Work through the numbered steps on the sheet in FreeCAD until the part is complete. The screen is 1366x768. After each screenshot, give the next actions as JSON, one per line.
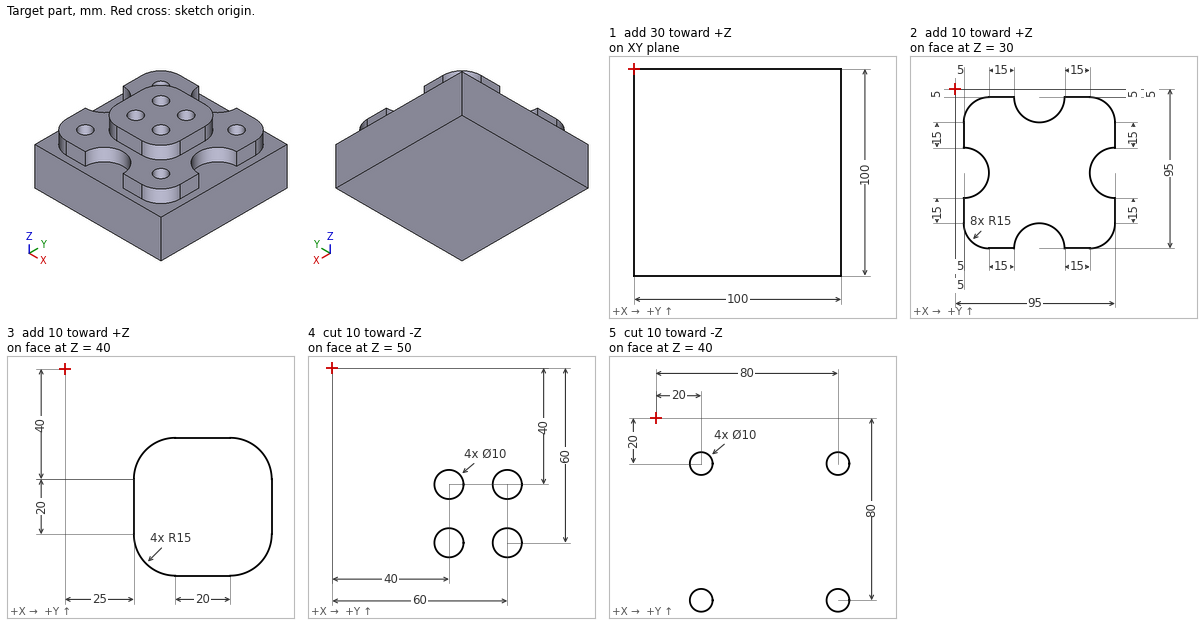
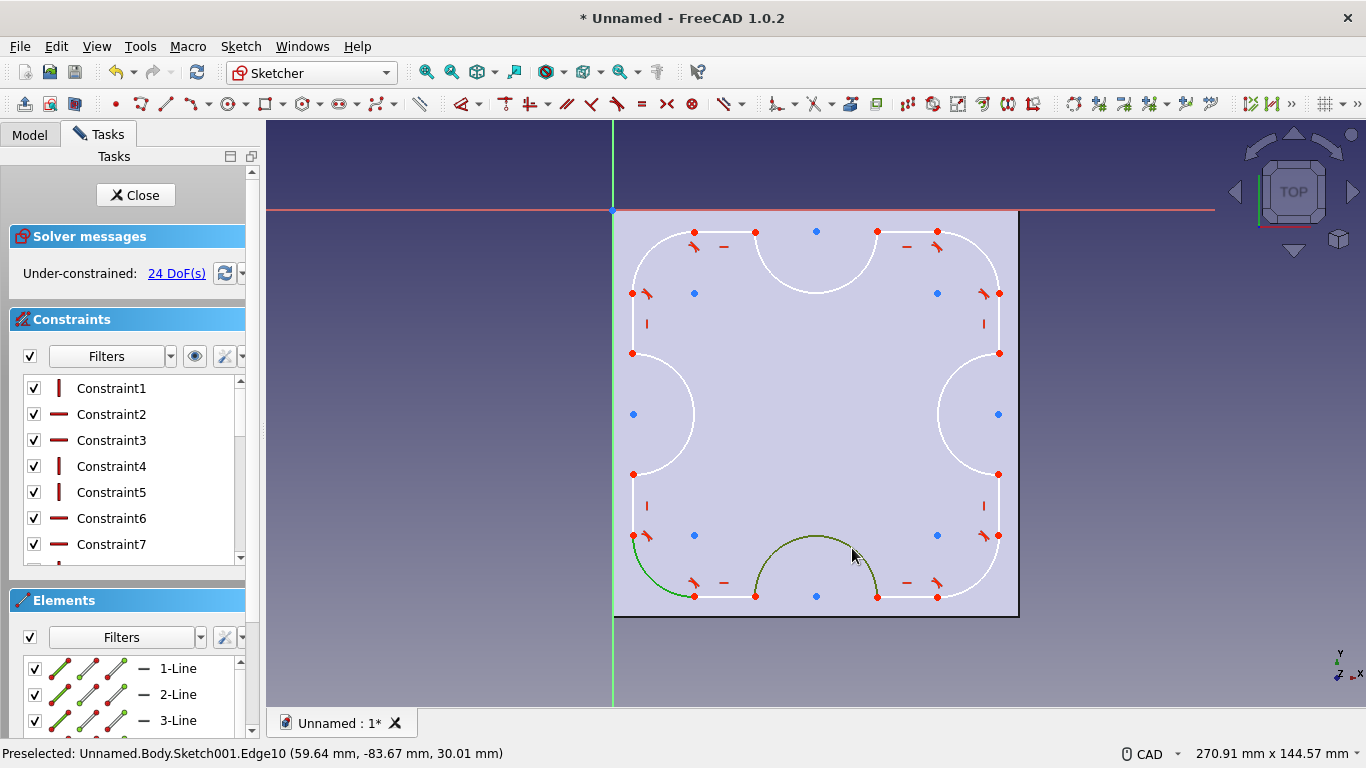
{"action": "left_click", "coordinate": [965, 591]}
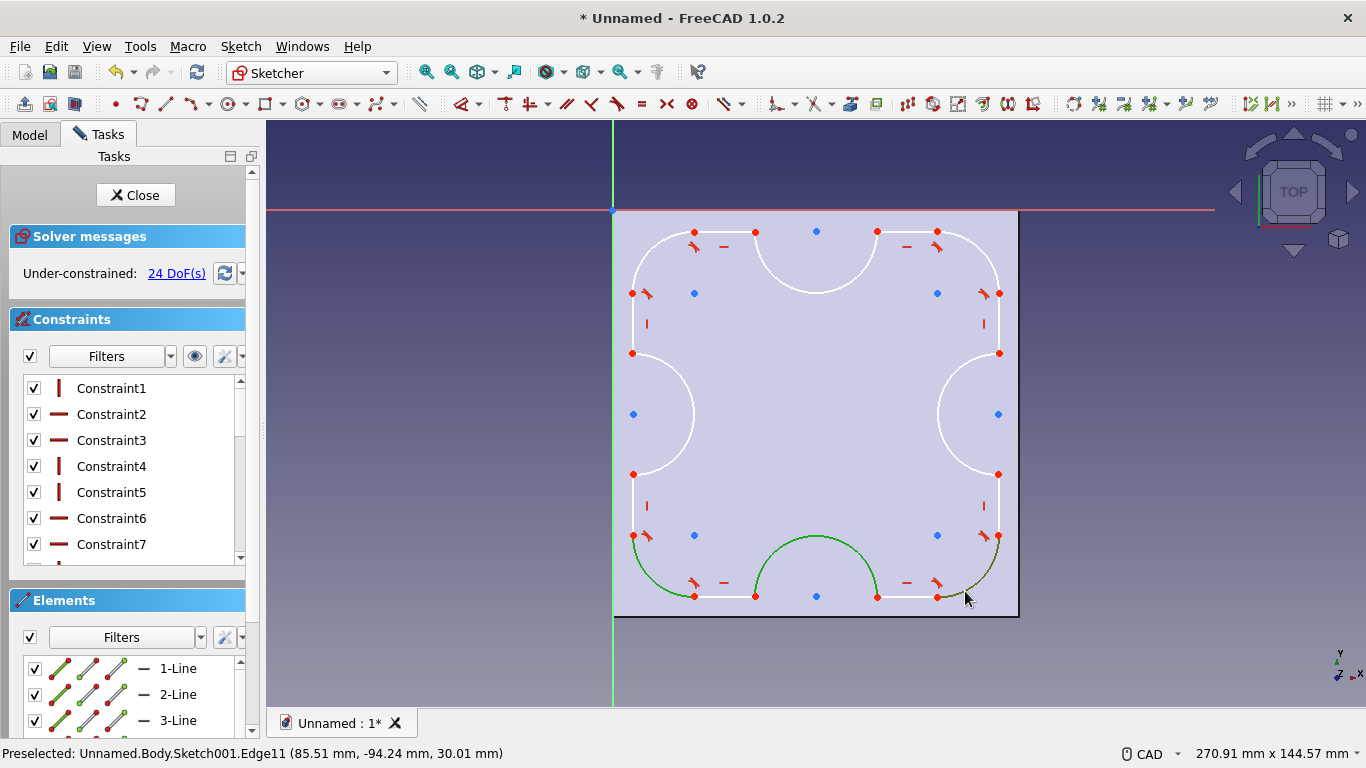
{"action": "left_click", "coordinate": [950, 379]}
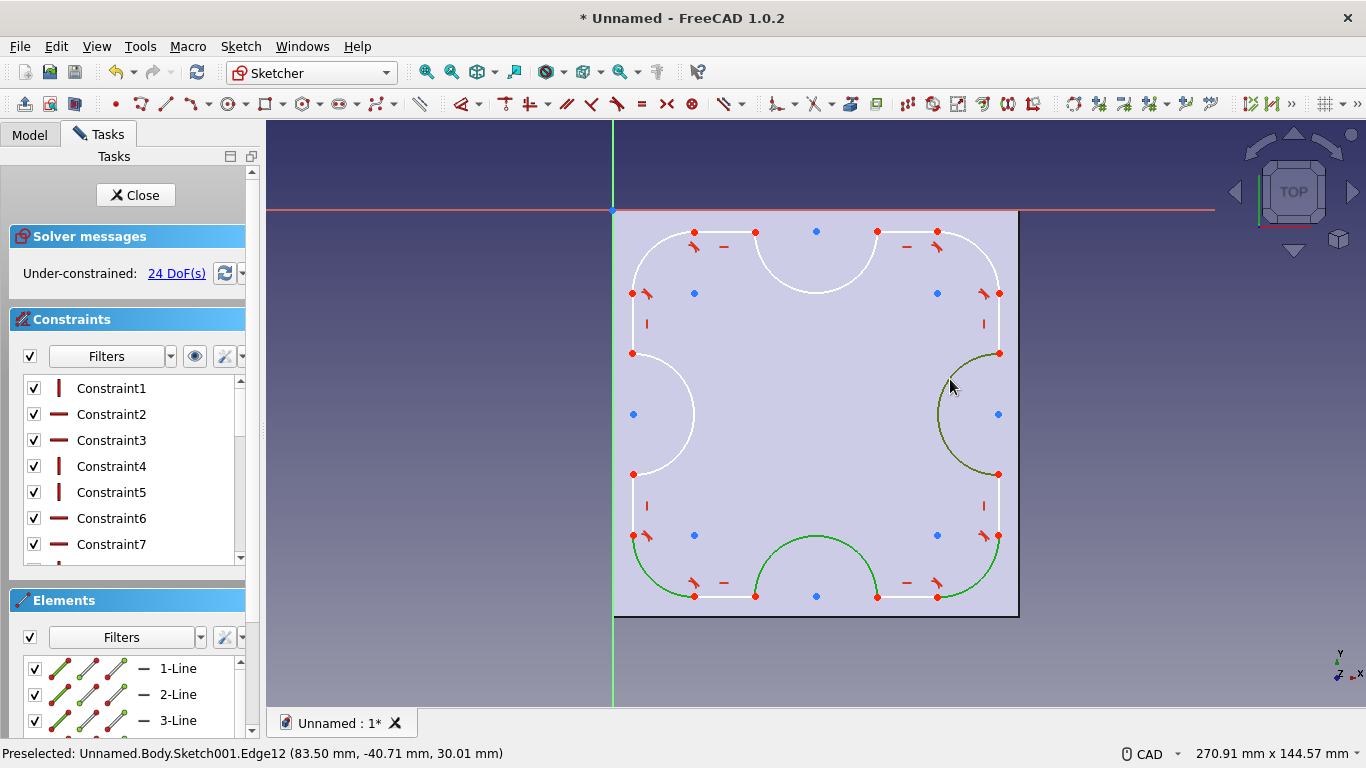
{"action": "left_click", "coordinate": [992, 266]}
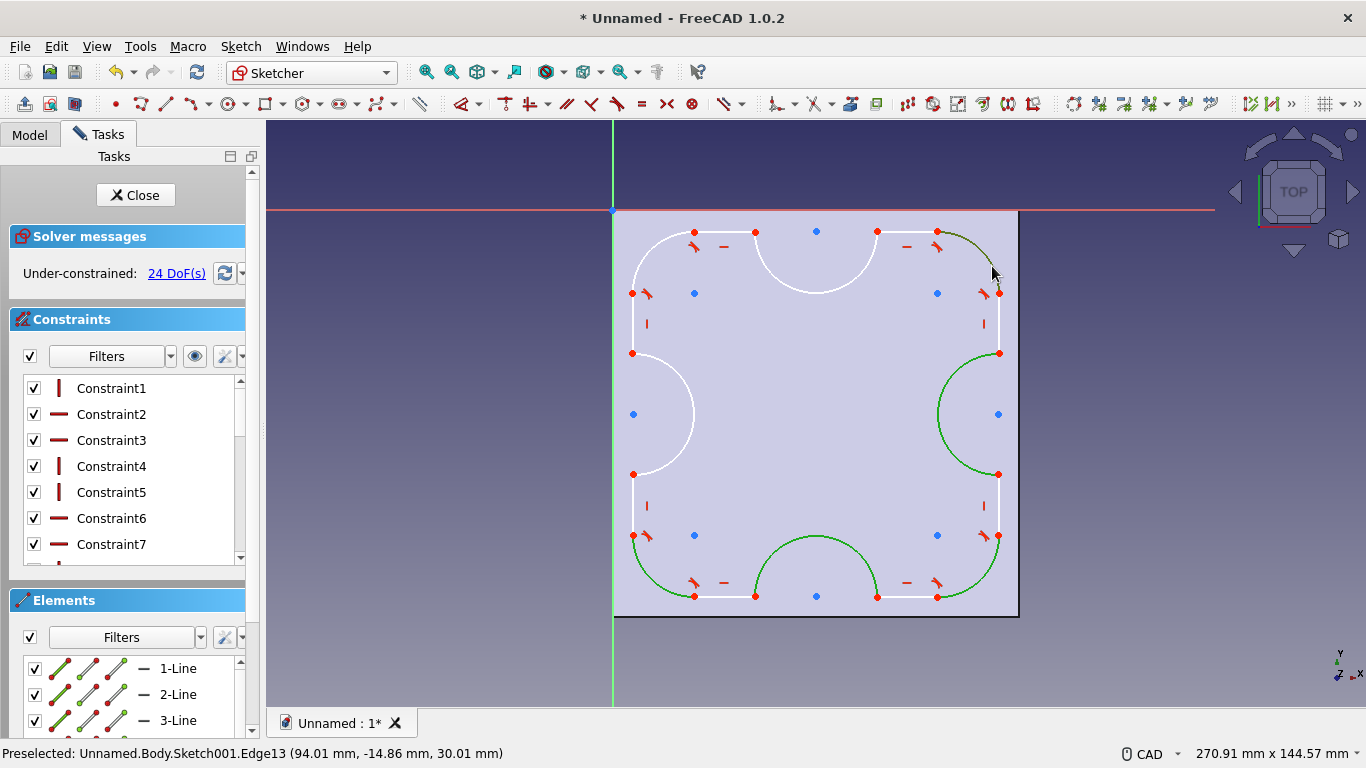
{"action": "left_click", "coordinate": [780, 281]}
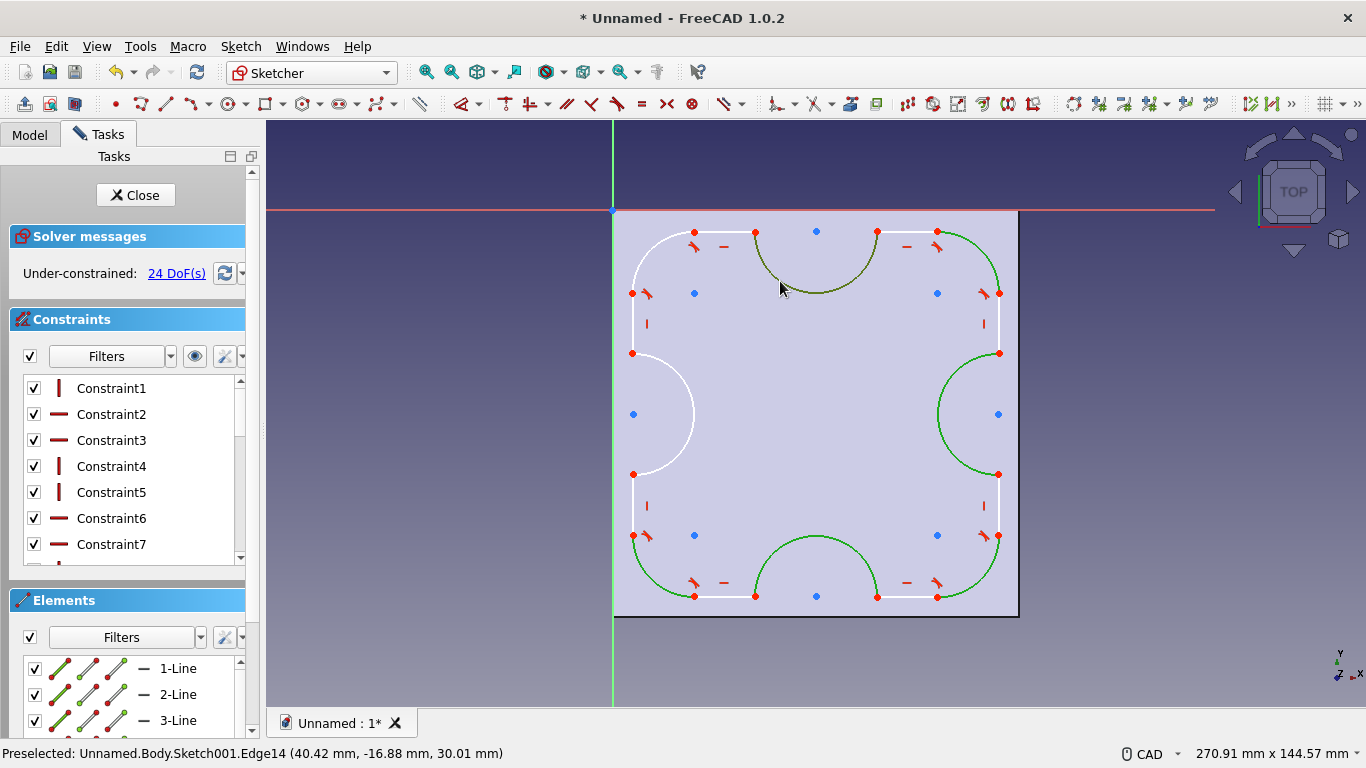
{"action": "left_click", "coordinate": [666, 239]}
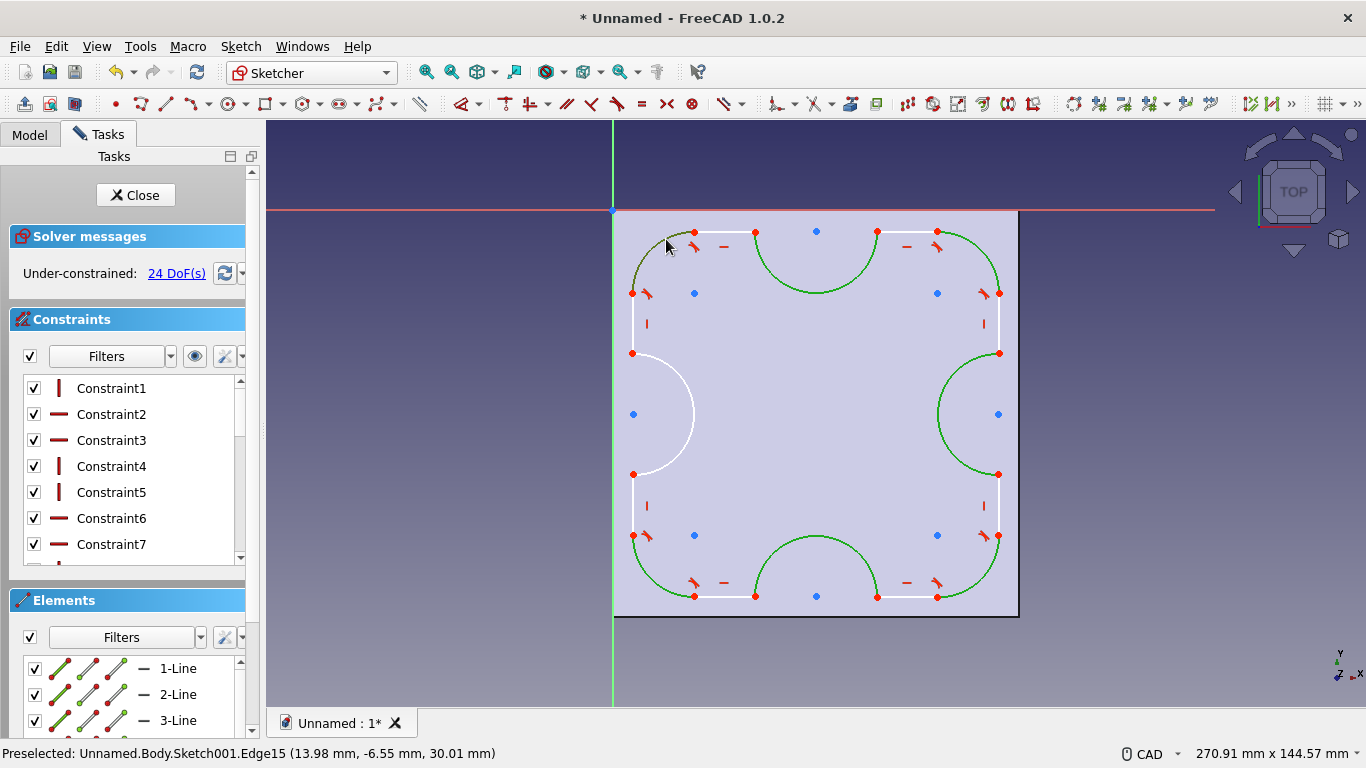
{"action": "left_click", "coordinate": [682, 450]}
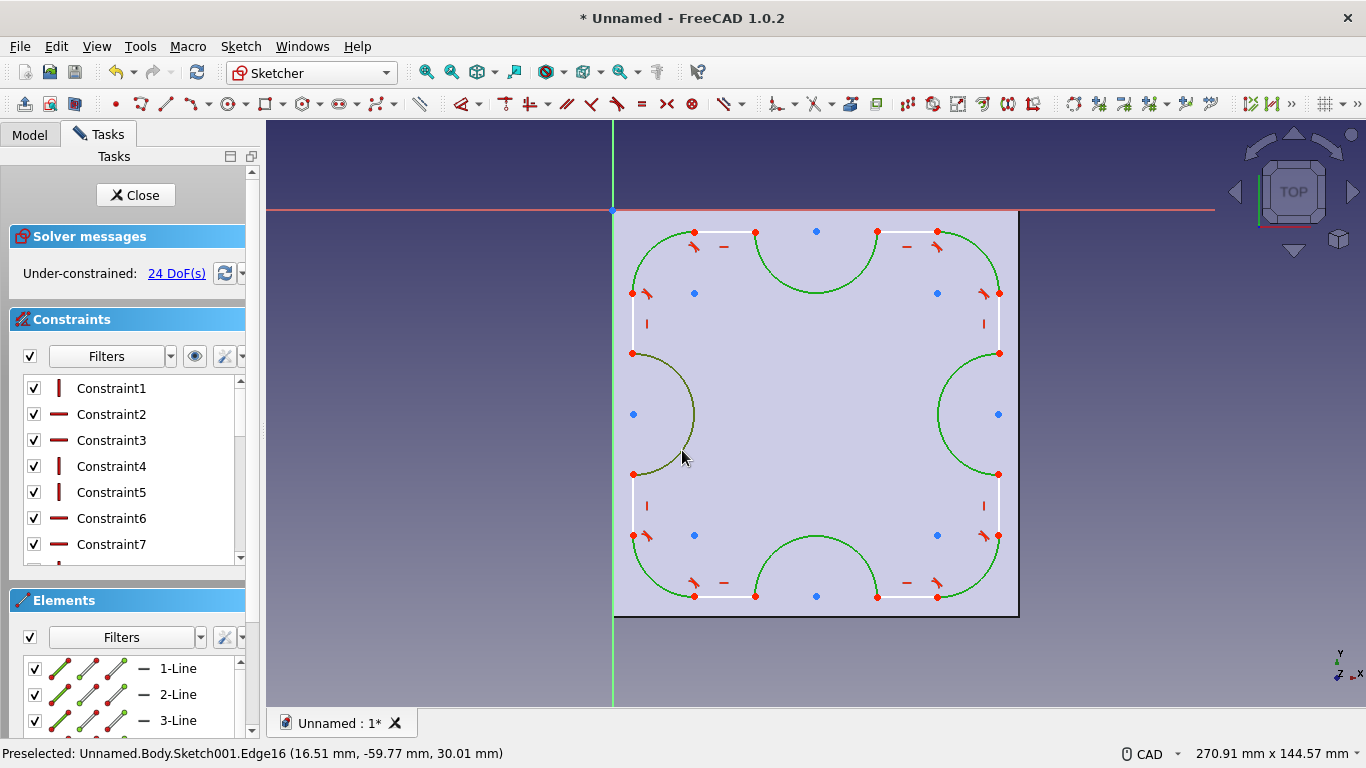
{"action": "left_click", "coordinate": [642, 104]}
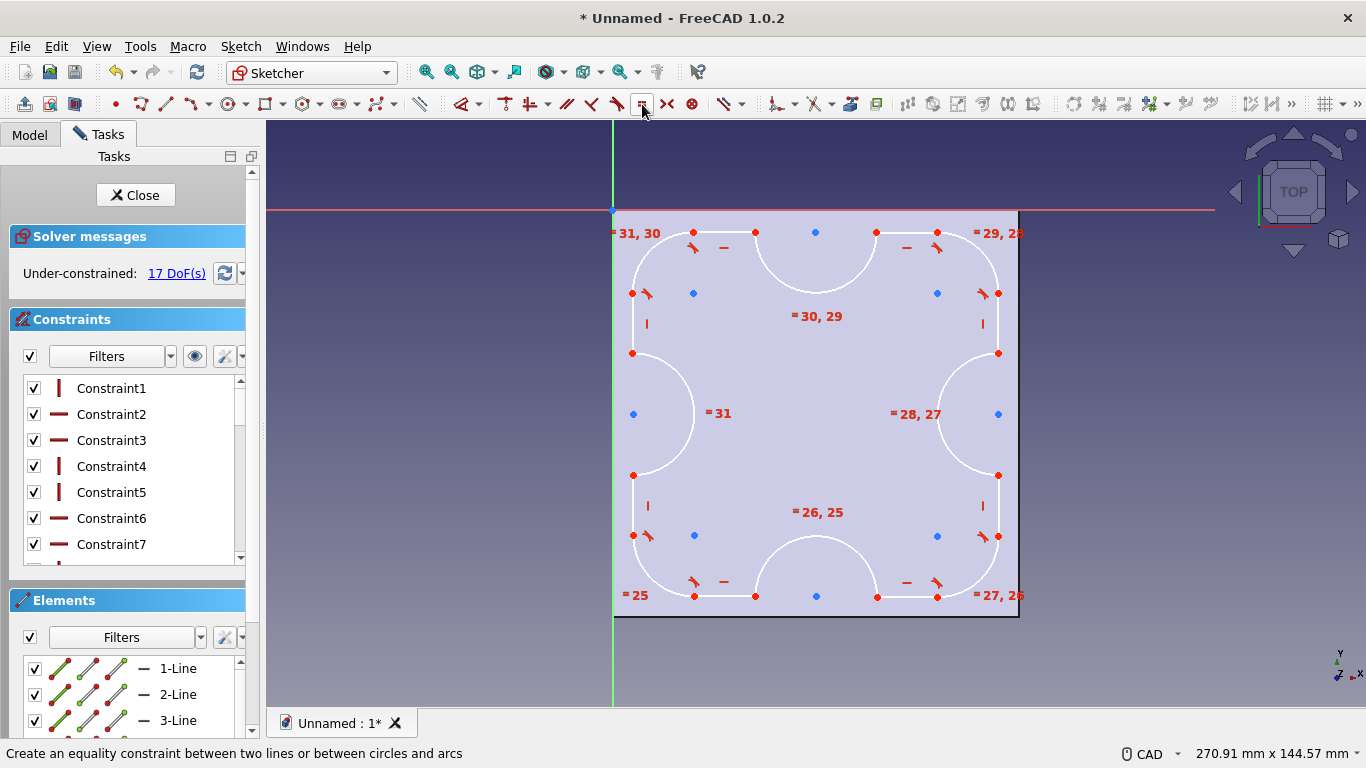
{"action": "left_click", "coordinate": [460, 104]}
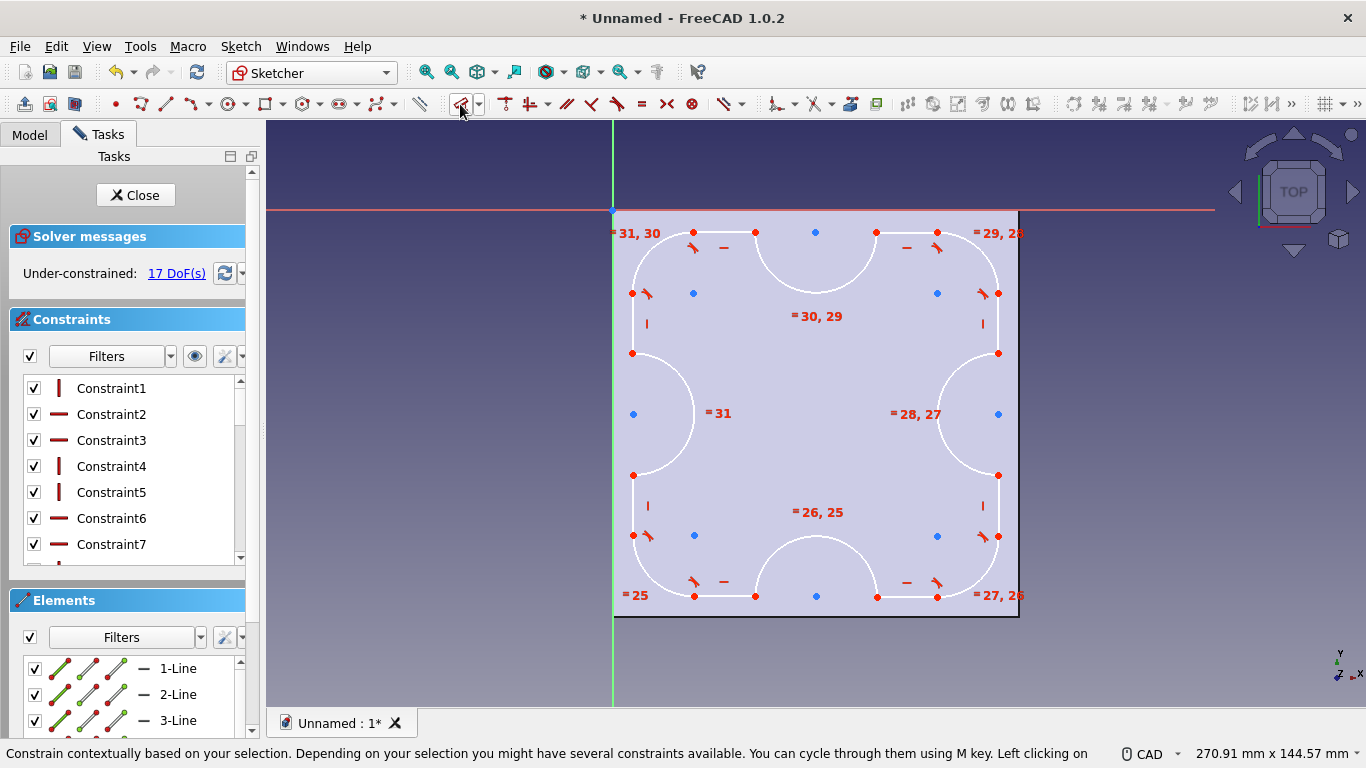
{"action": "left_click", "coordinate": [640, 563]}
{"action": "left_click", "coordinate": [642, 612]}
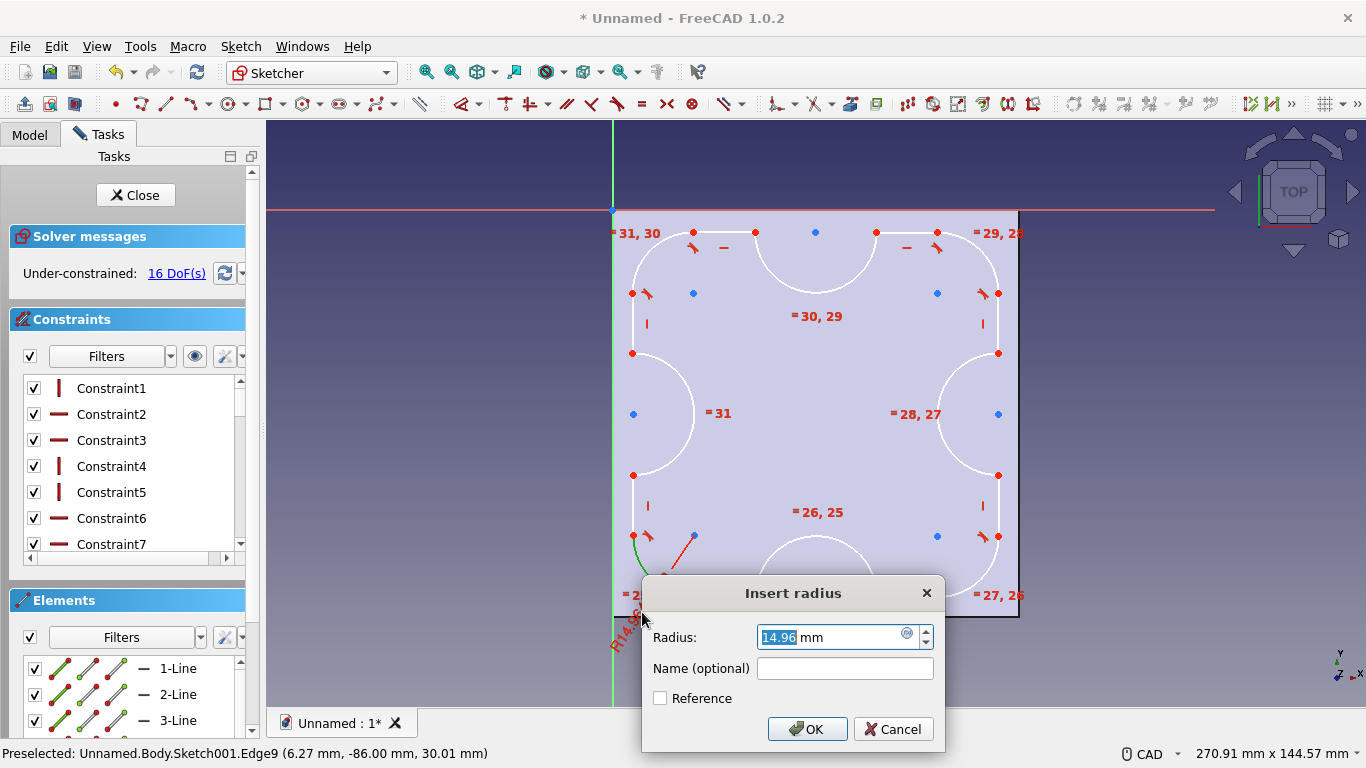
{"action": "type", "text": "15"}
{"action": "key", "text": "Return"}